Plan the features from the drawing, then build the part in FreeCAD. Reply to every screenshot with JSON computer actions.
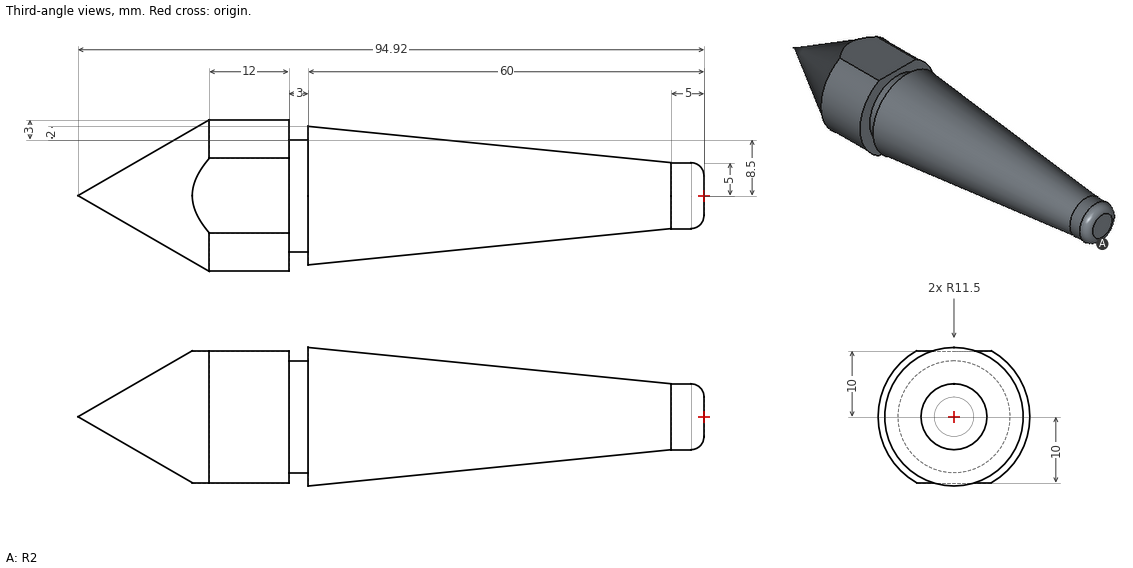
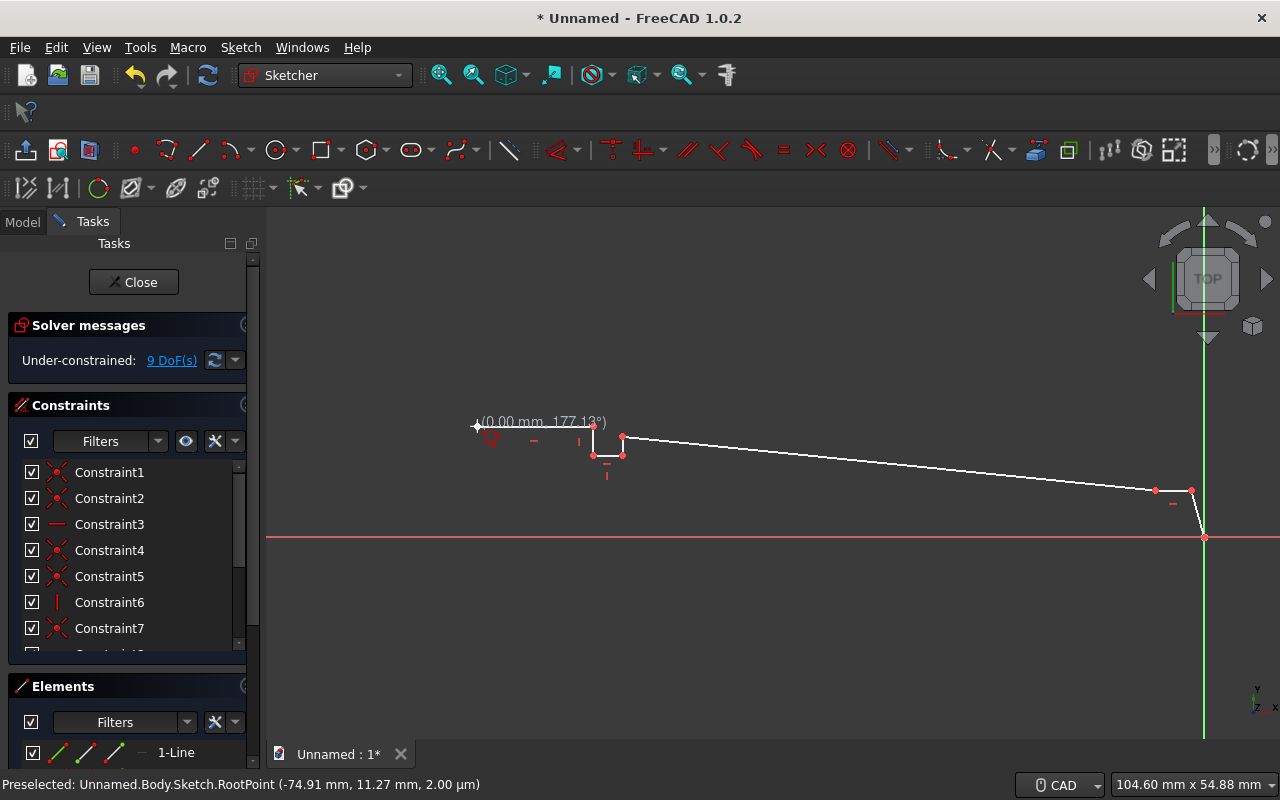
{"action": "scroll", "coordinate": [624, 456], "scroll_direction": "down", "scroll_amount": 2}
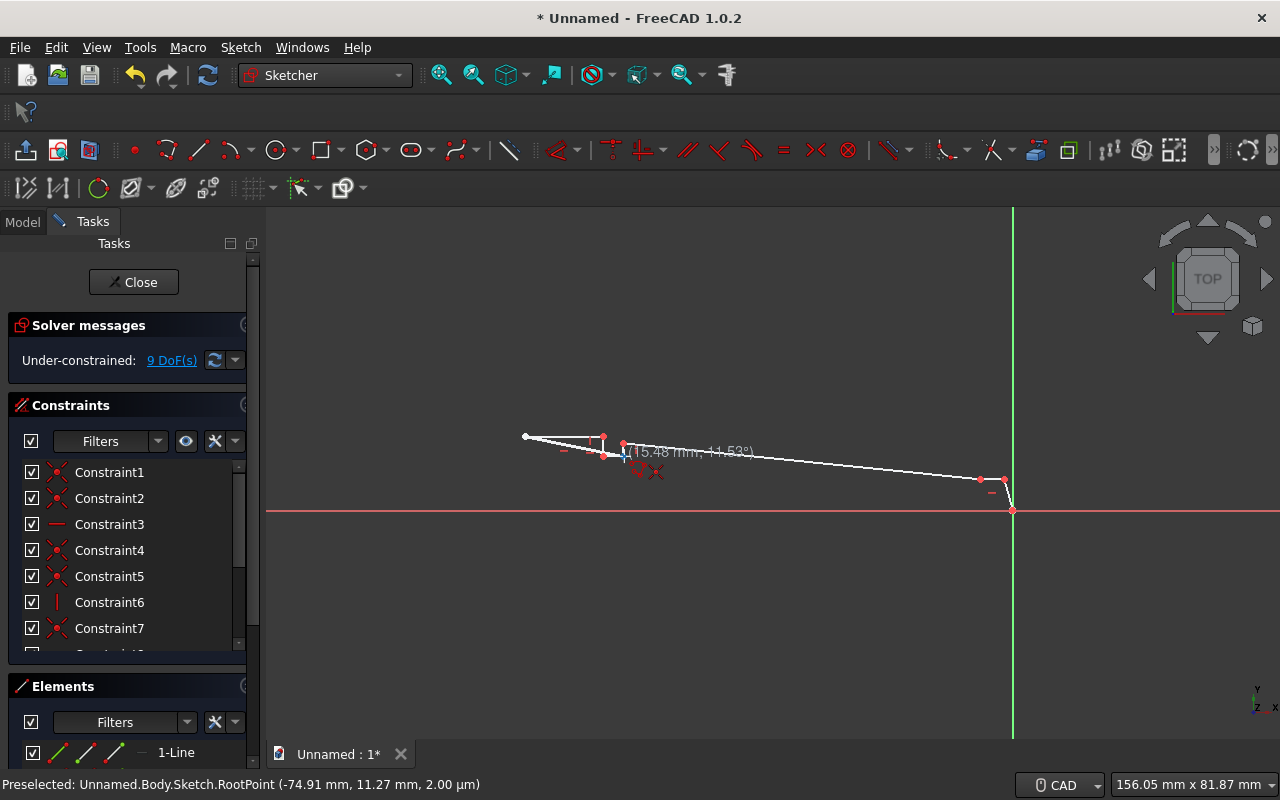
{"action": "left_click", "coordinate": [396, 502]}
{"action": "left_click", "coordinate": [1013, 511]}
{"action": "key", "text": "Escape"}
{"action": "key", "text": "Escape"}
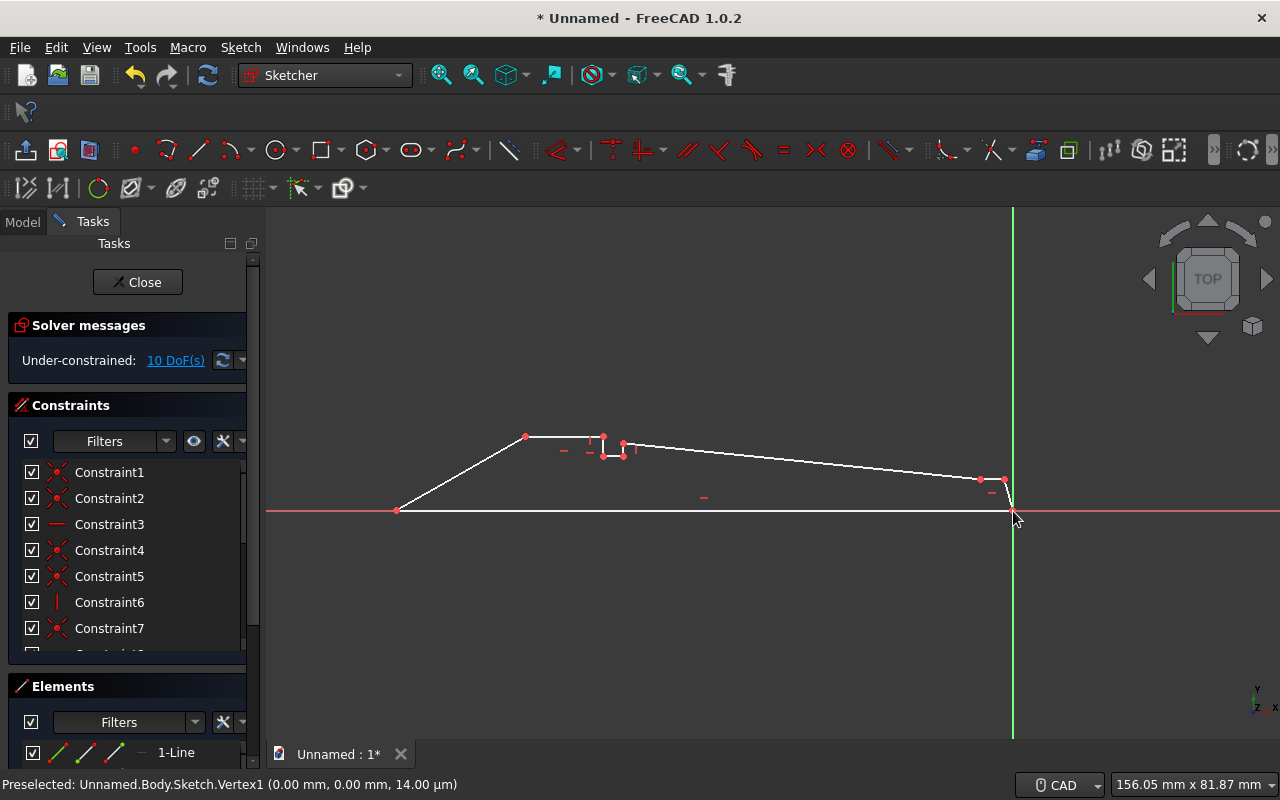
{"action": "scroll", "coordinate": [1010, 501], "scroll_direction": "up", "scroll_amount": 2}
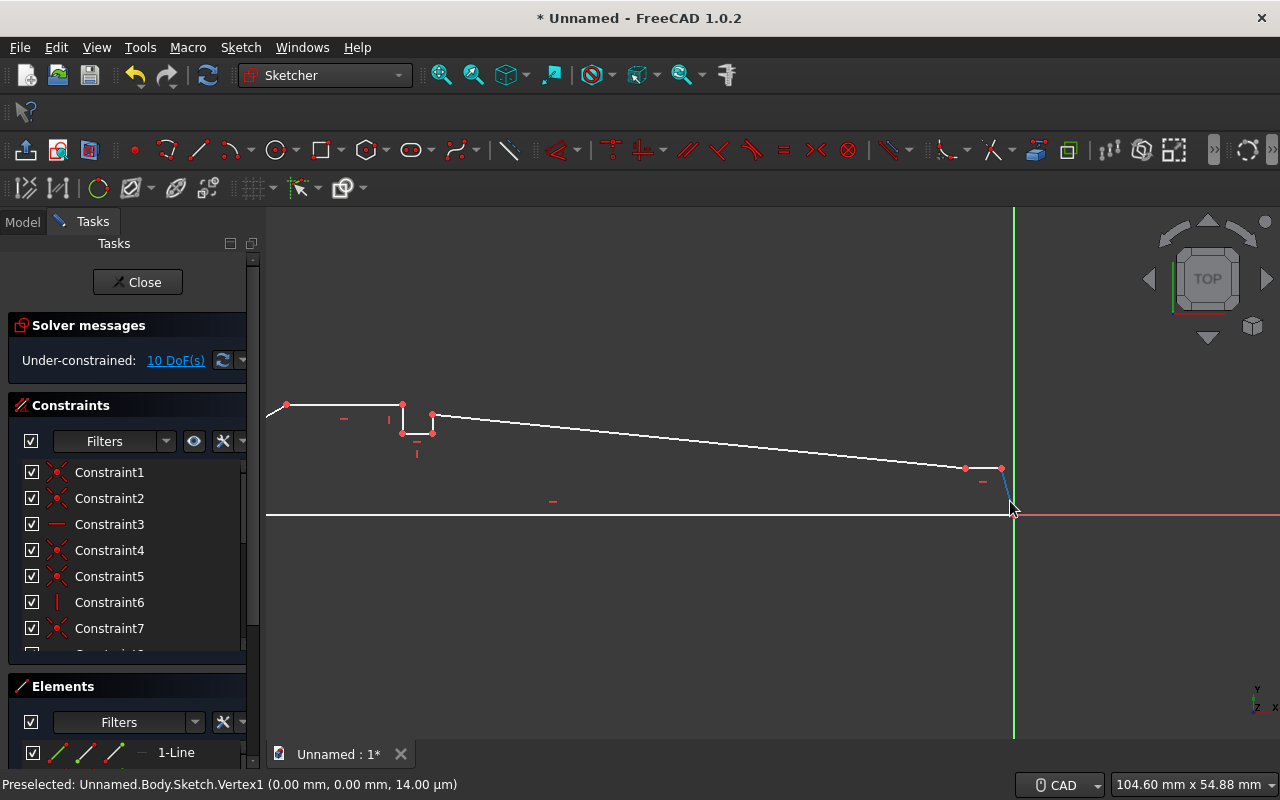
{"action": "left_click", "coordinate": [1010, 501]}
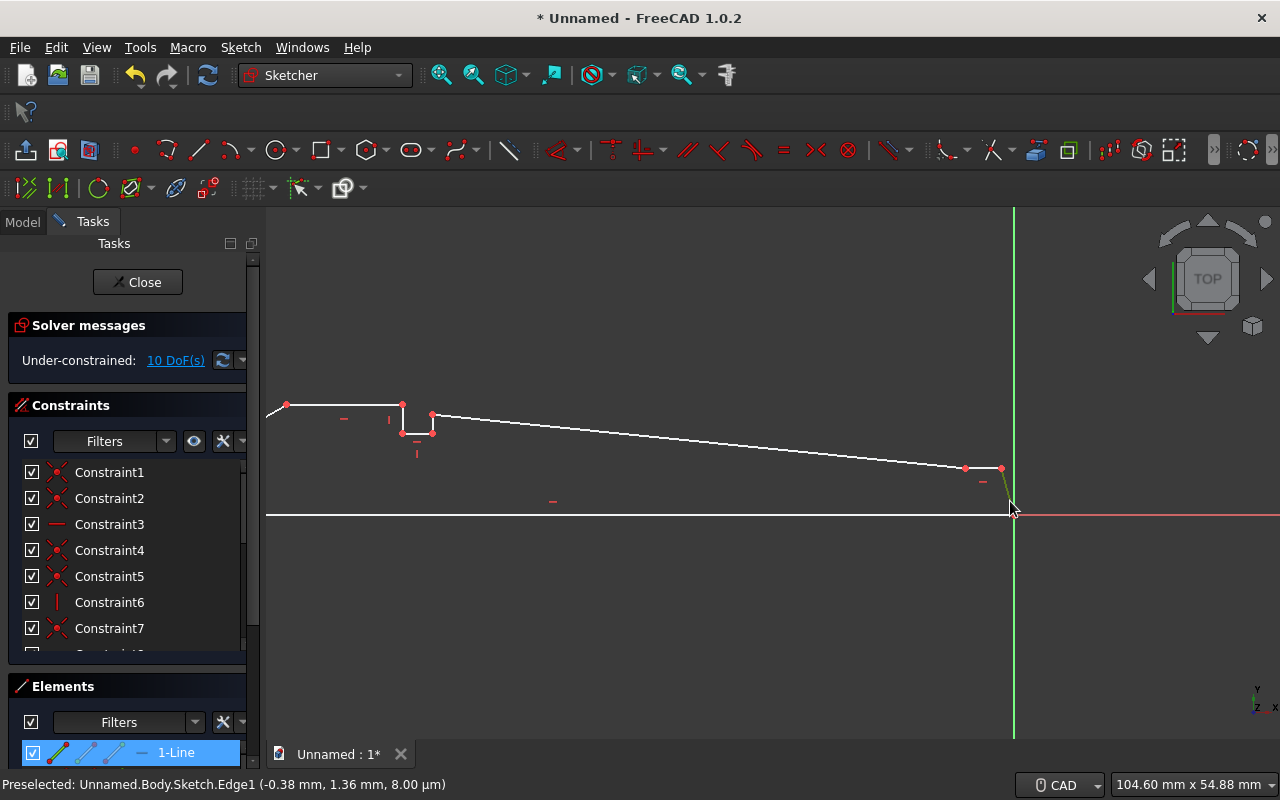
{"action": "key", "text": "v"}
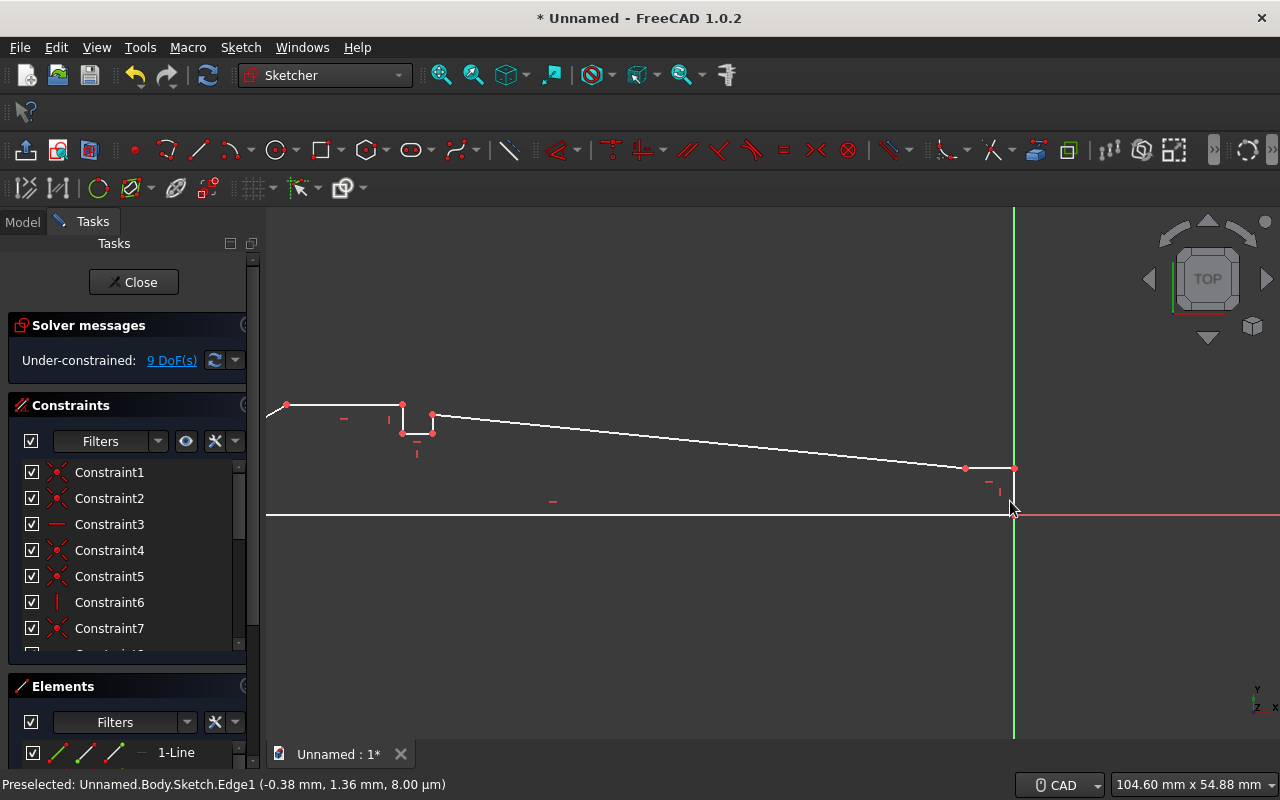
{"action": "left_click", "coordinate": [556, 150]}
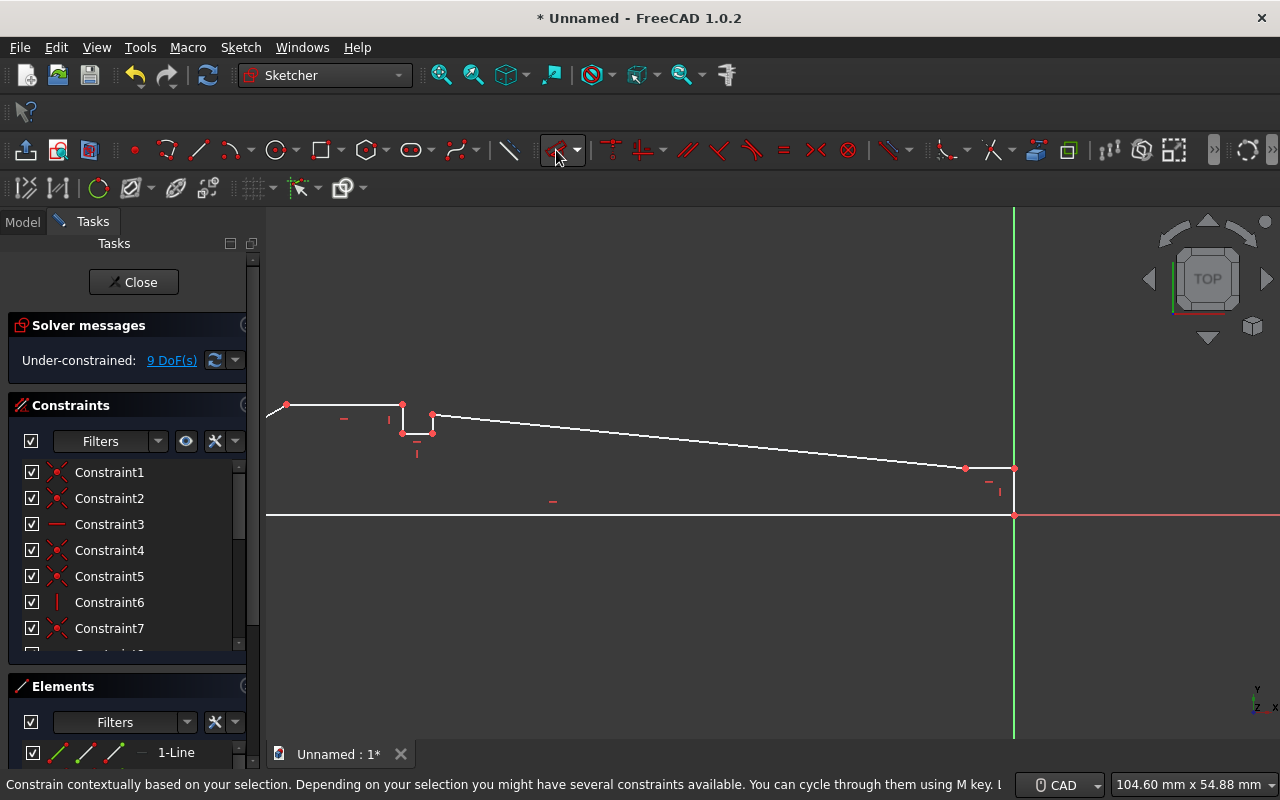
{"action": "left_click", "coordinate": [1014, 501]}
{"action": "left_click", "coordinate": [1048, 492]}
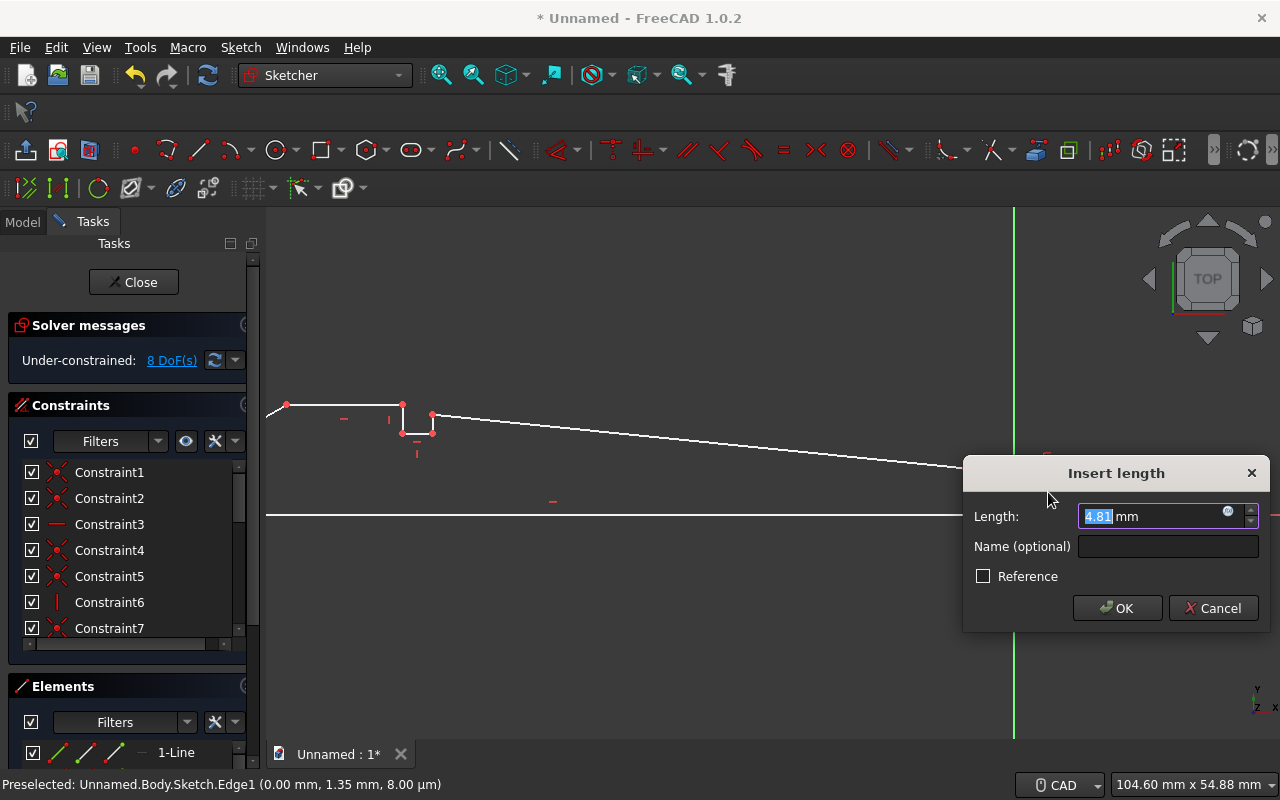
{"action": "type", "text": "5"}
{"action": "key", "text": "Return"}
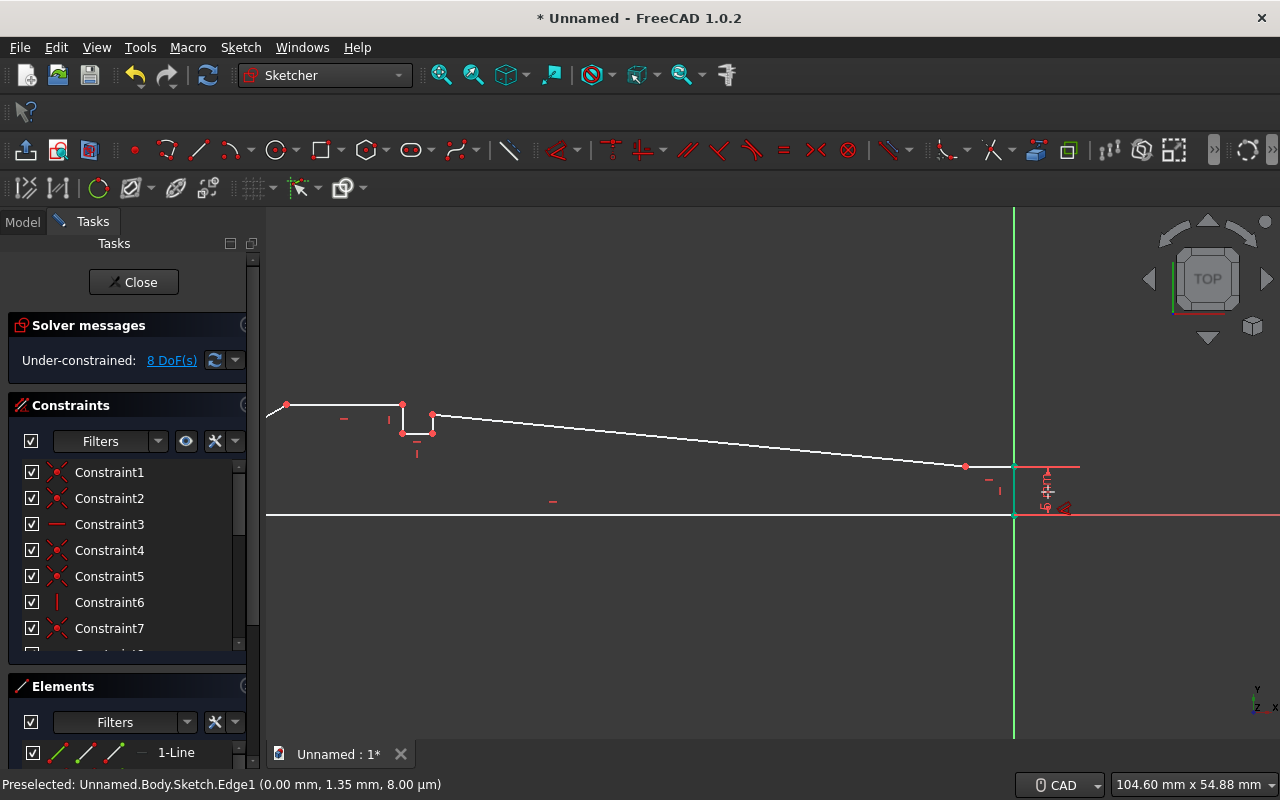
{"action": "left_click", "coordinate": [999, 467]}
{"action": "left_click", "coordinate": [973, 501]}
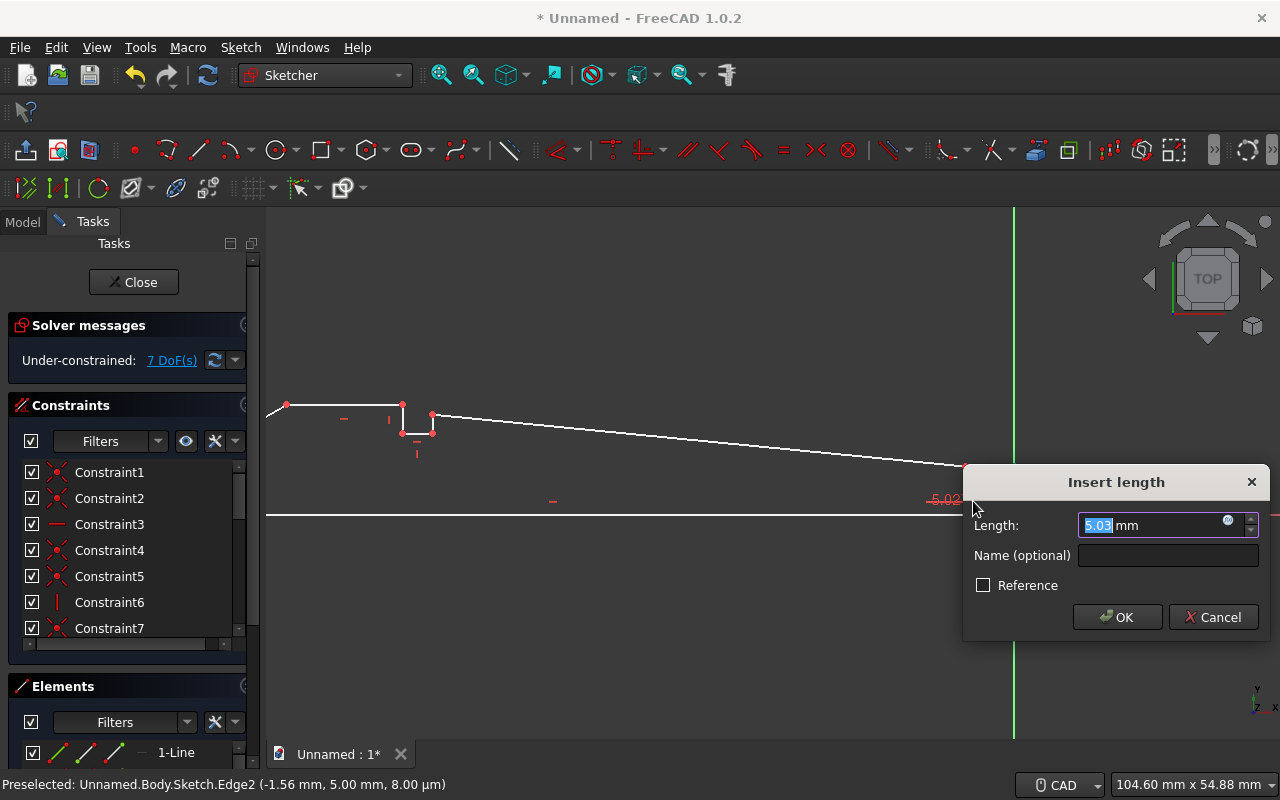
{"action": "type", "text": "5"}
{"action": "key", "text": "Return"}